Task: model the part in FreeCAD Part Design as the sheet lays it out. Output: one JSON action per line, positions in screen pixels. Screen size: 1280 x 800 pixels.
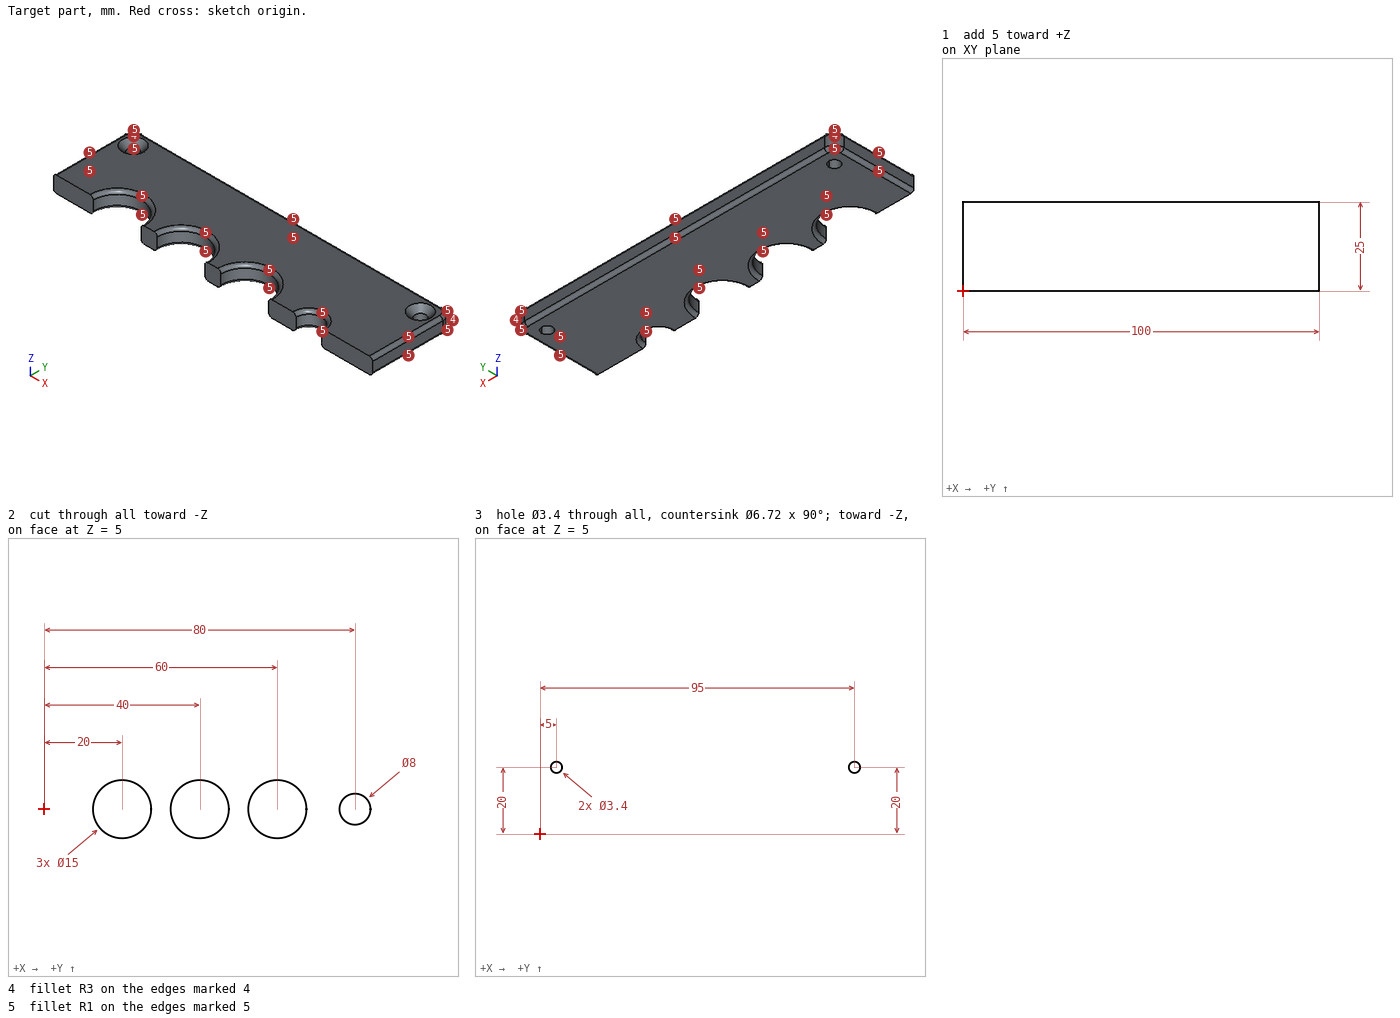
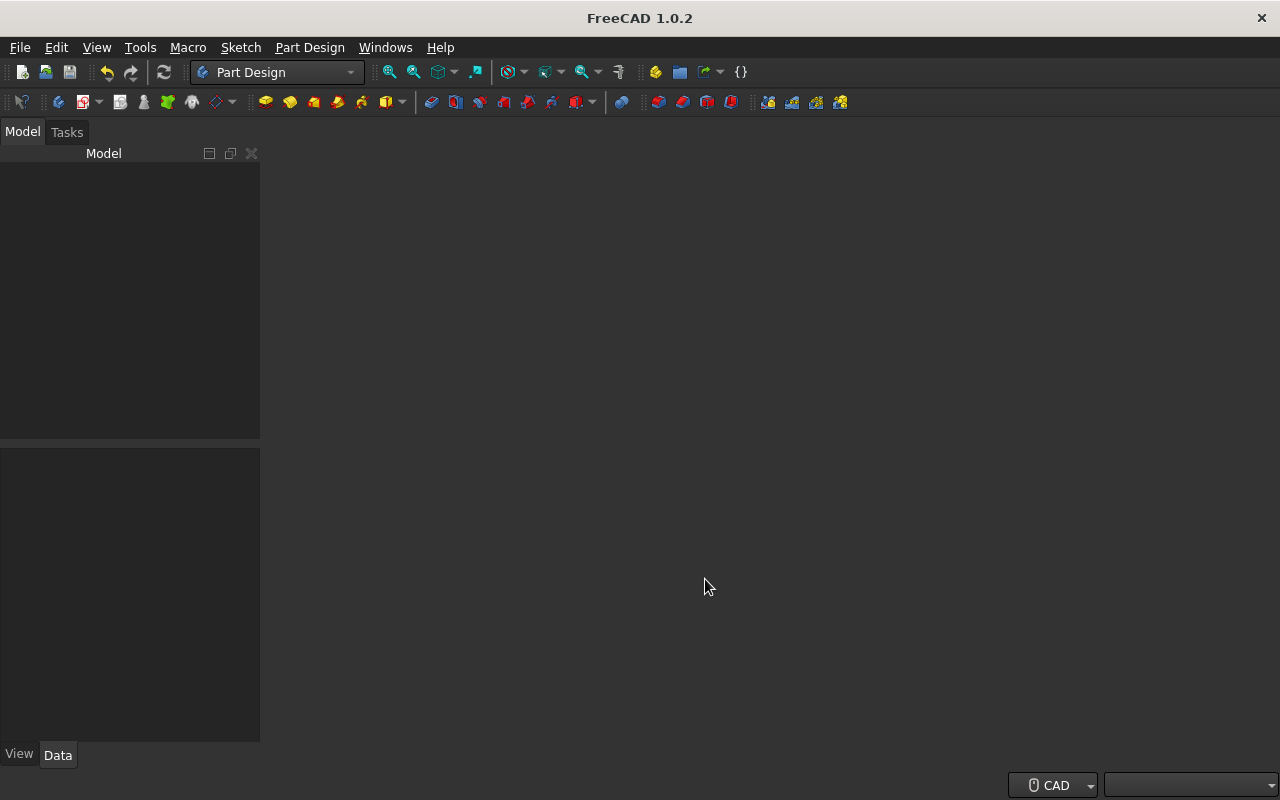
{"action": "left_click", "coordinate": [22, 72]}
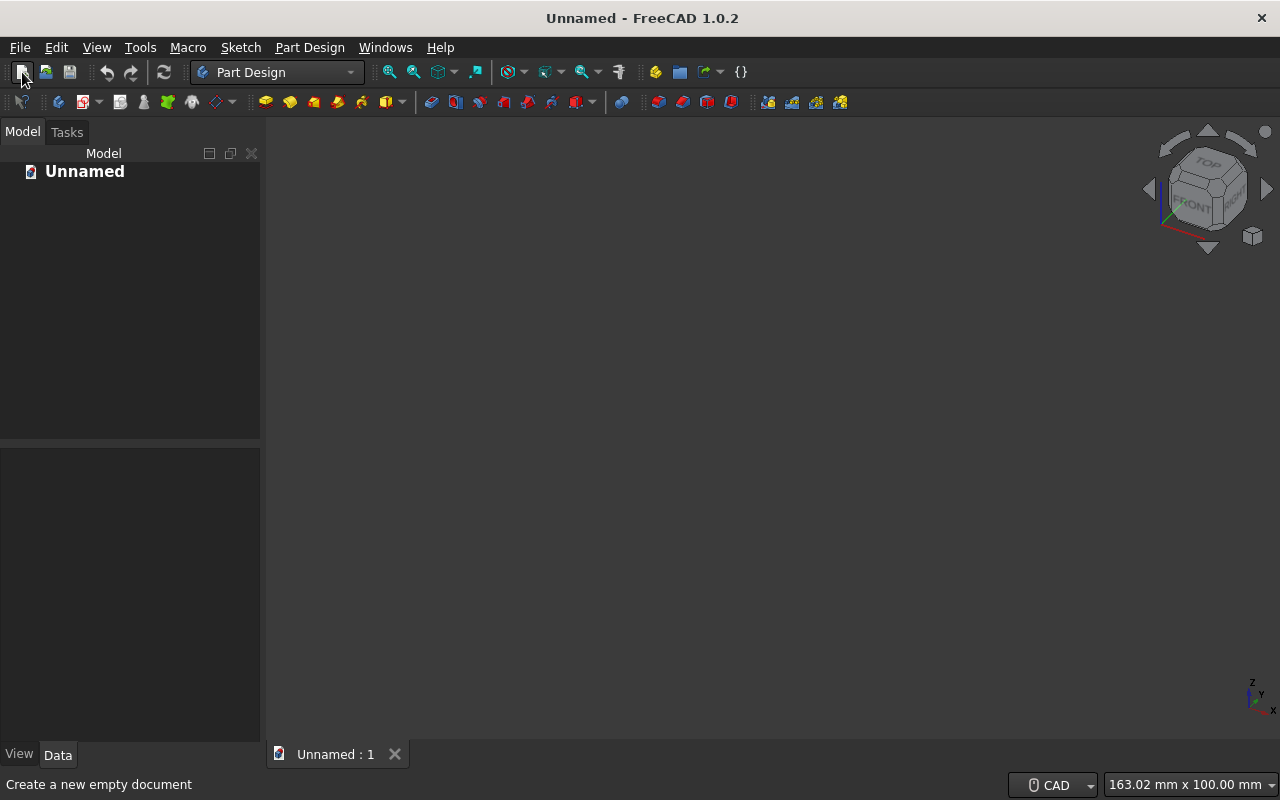
{"action": "left_click", "coordinate": [84, 102]}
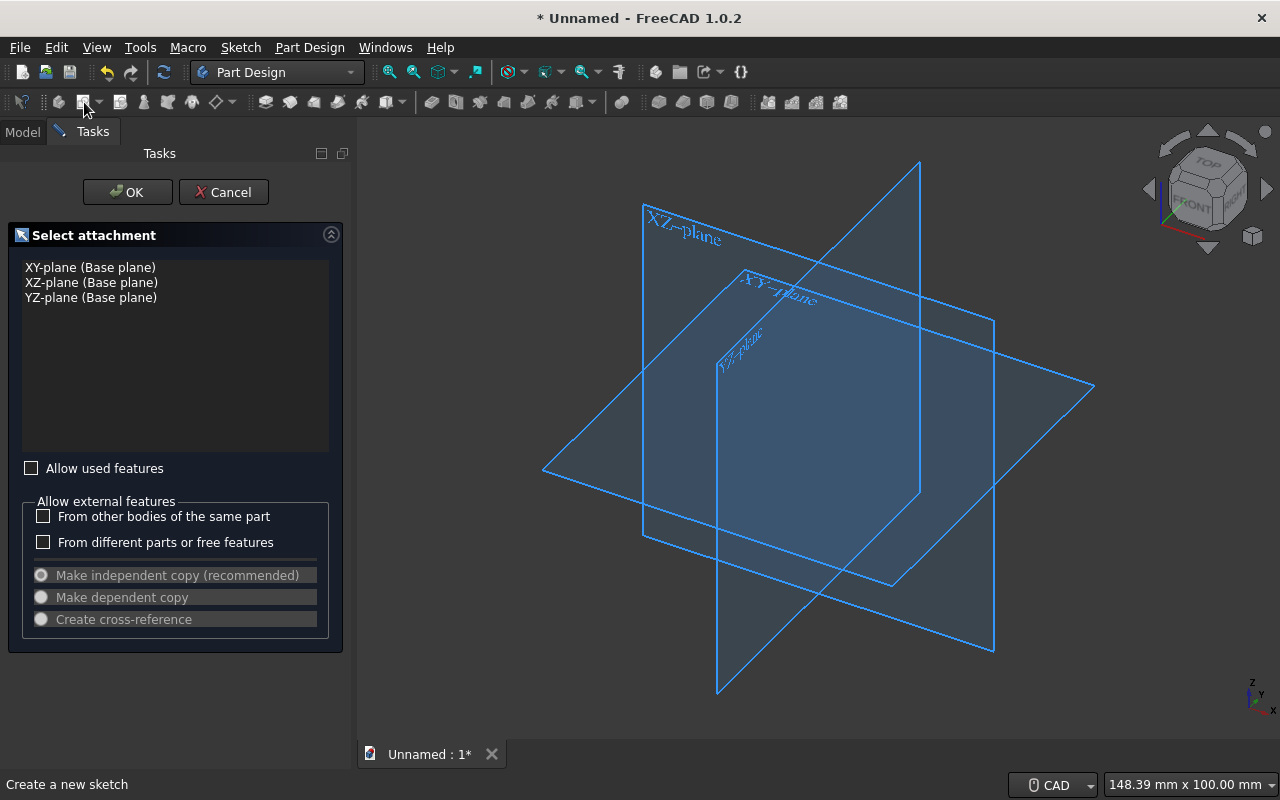
{"action": "left_click", "coordinate": [82, 268]}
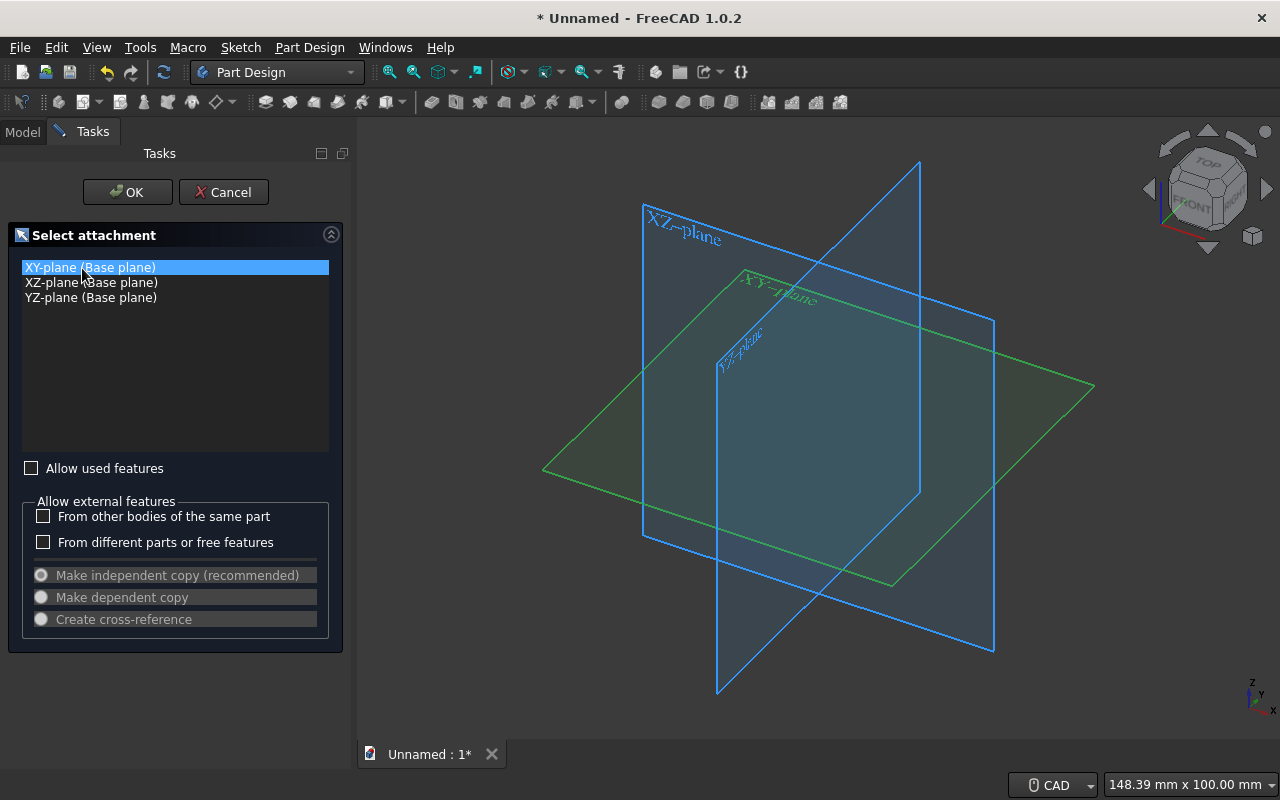
{"action": "left_click", "coordinate": [128, 192]}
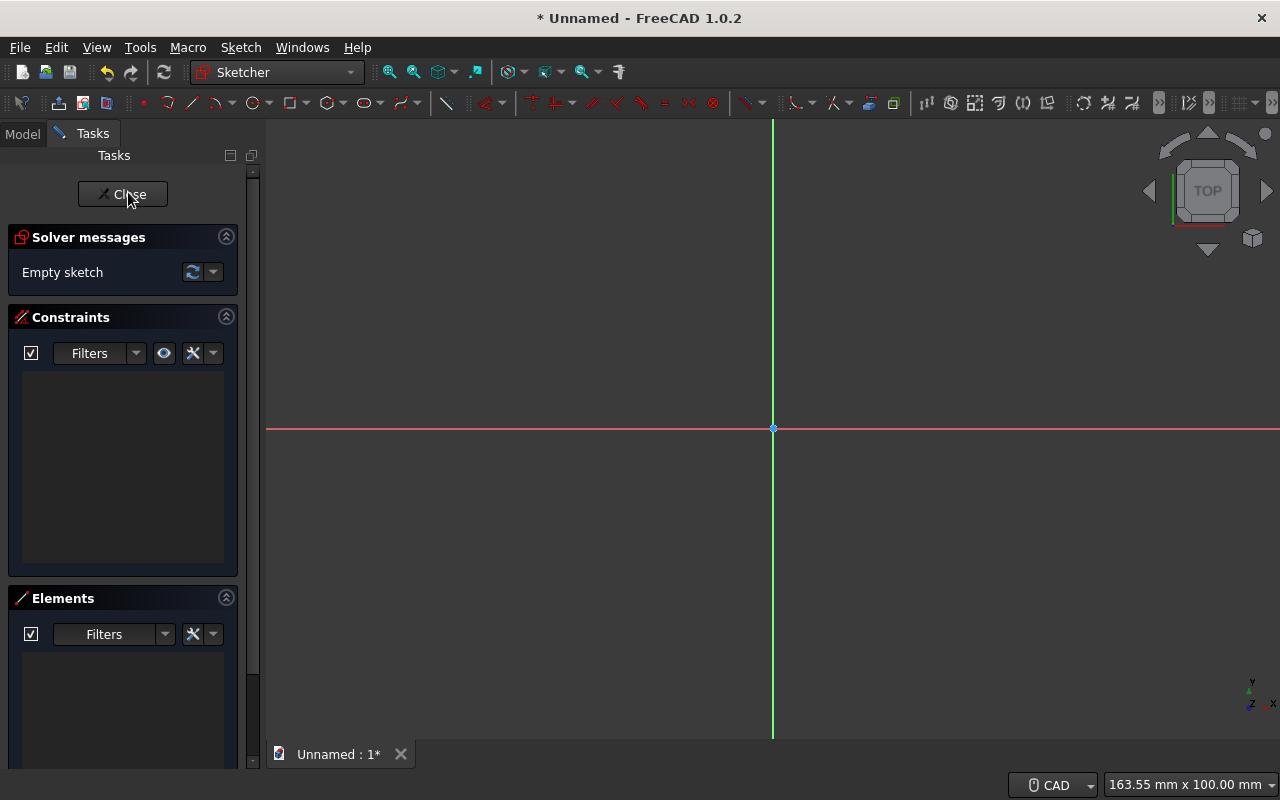
{"action": "scroll", "coordinate": [294, 587], "scroll_direction": "down", "scroll_amount": 2}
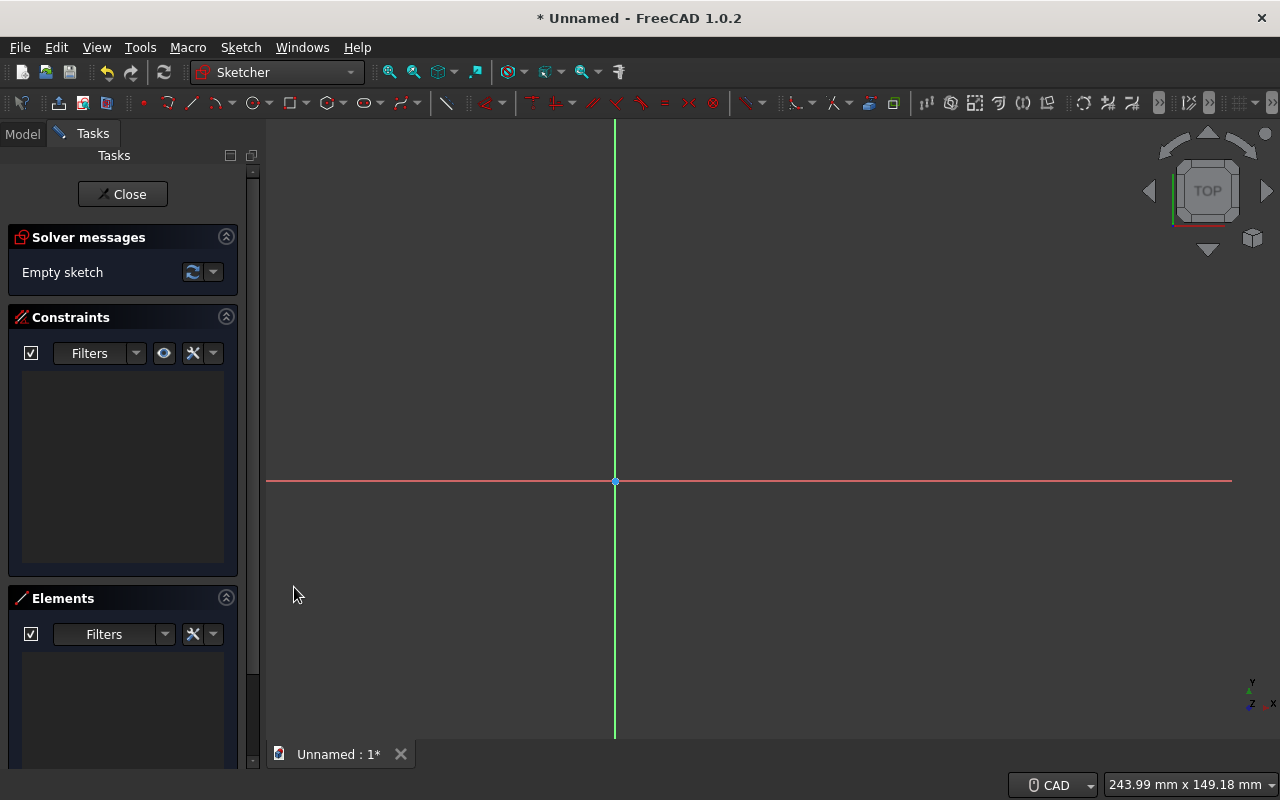
{"action": "scroll", "coordinate": [1064, 430], "scroll_direction": "up", "scroll_amount": 2}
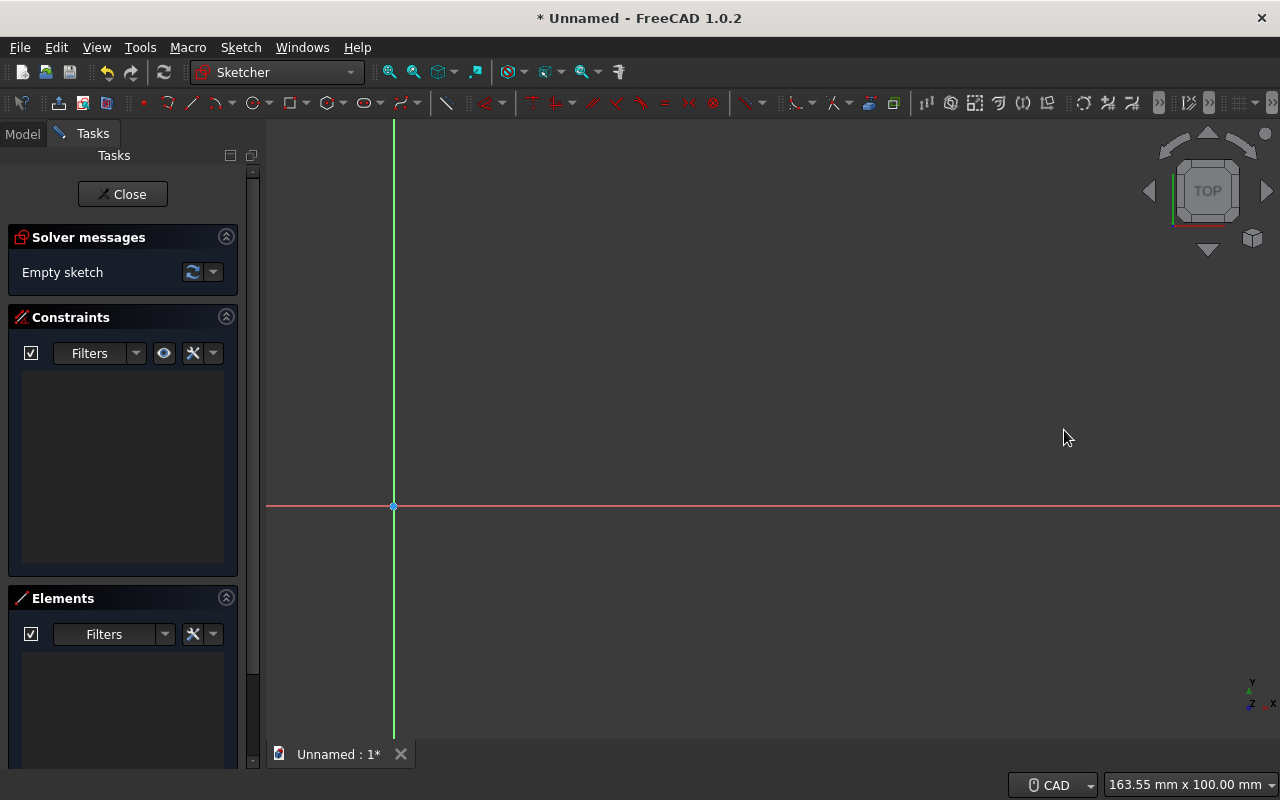
{"action": "left_click", "coordinate": [290, 104]}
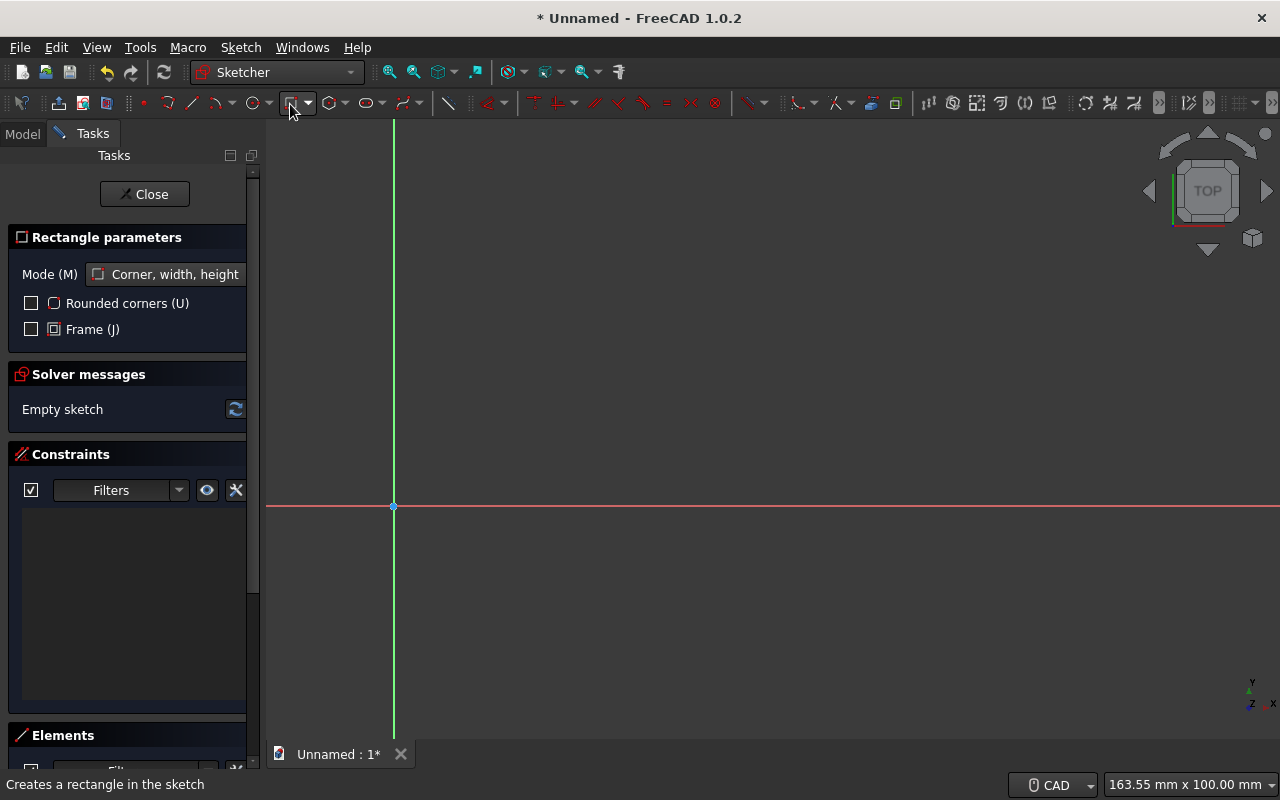
{"action": "left_click", "coordinate": [394, 506]}
{"action": "mouse_move", "coordinate": [1014, 351]}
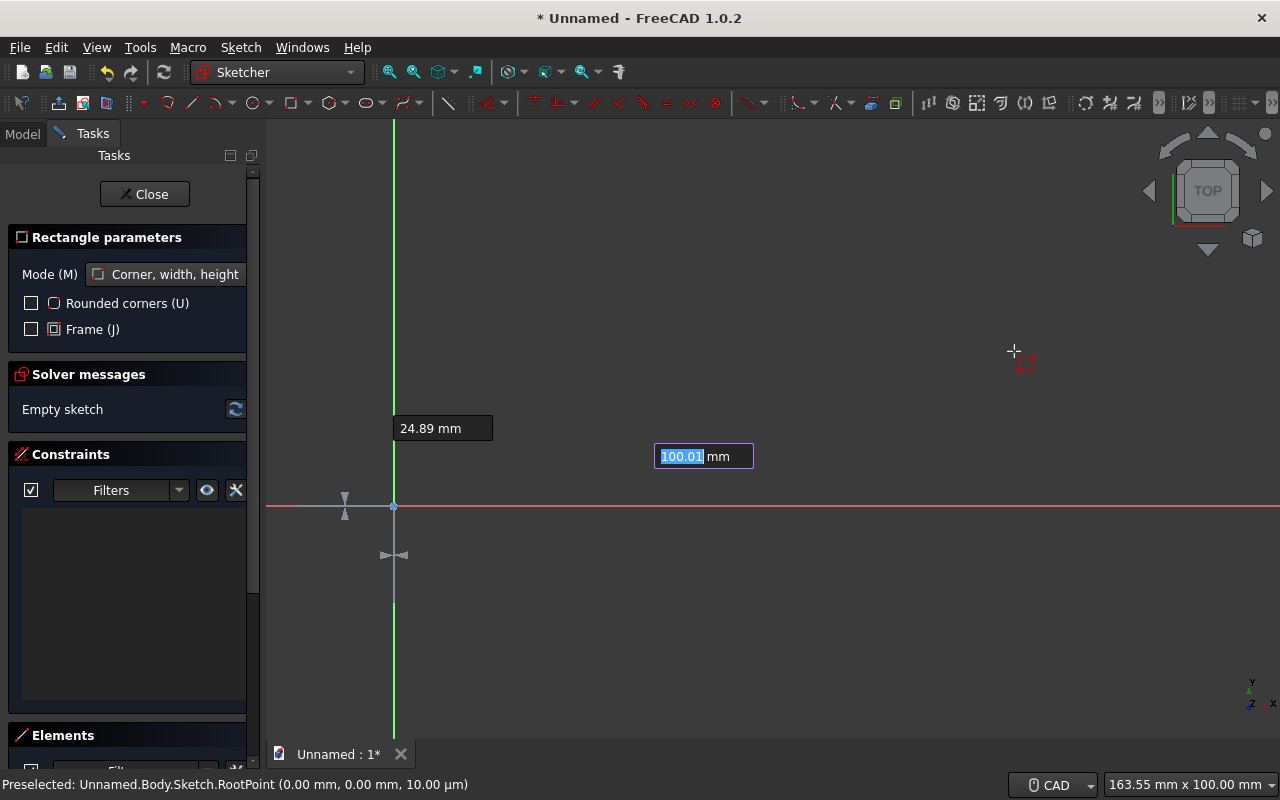
{"action": "type", "text": "100"}
{"action": "key", "text": "Tab"}
{"action": "type", "text": "25"}
{"action": "key", "text": "Return"}
{"action": "key", "text": "Escape"}